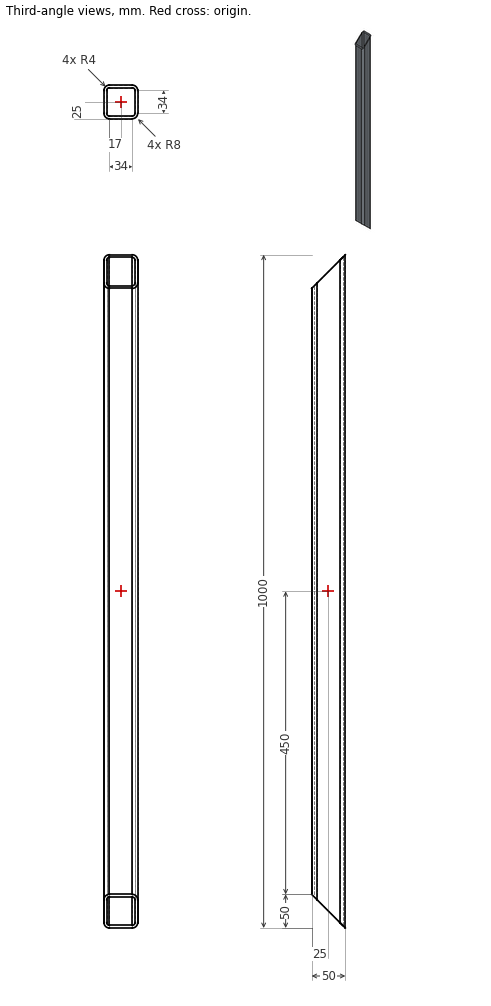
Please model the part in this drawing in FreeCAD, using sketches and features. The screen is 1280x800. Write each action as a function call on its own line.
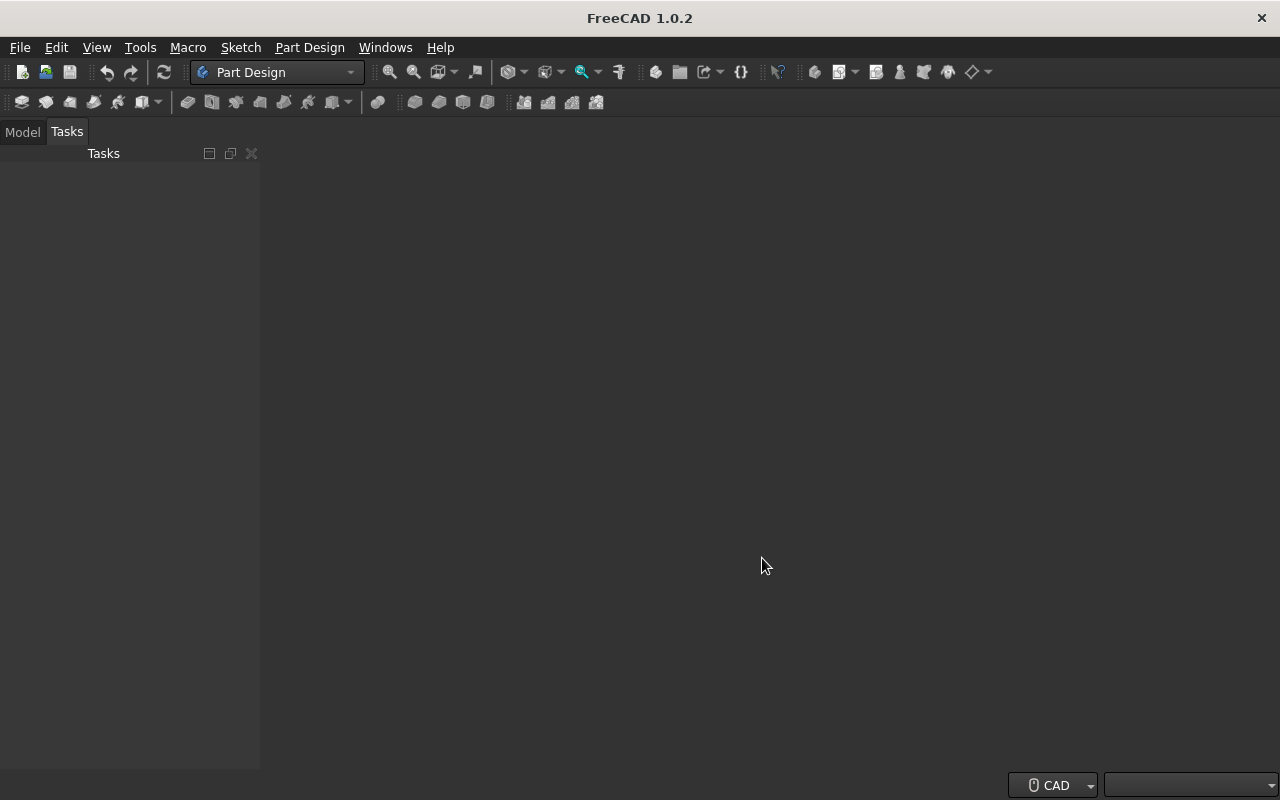
click(22, 72)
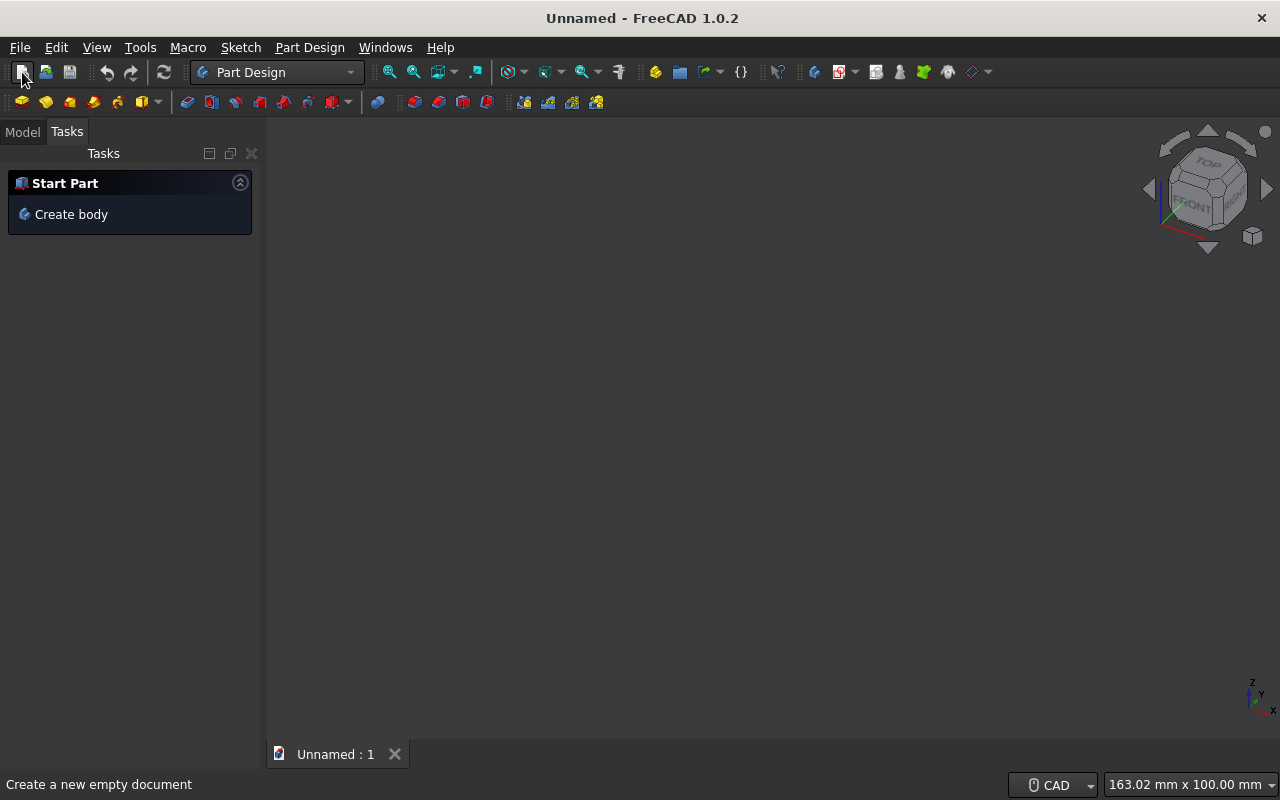
click(840, 72)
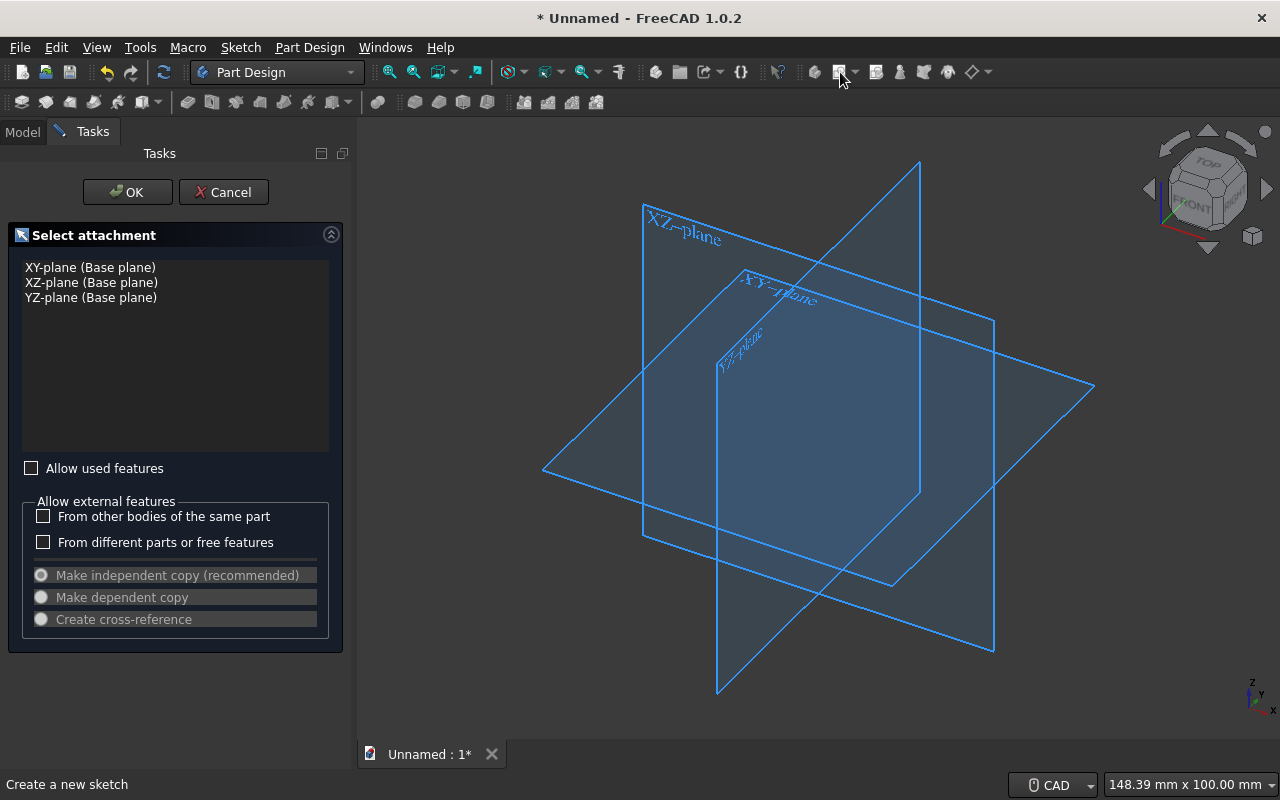
click(82, 268)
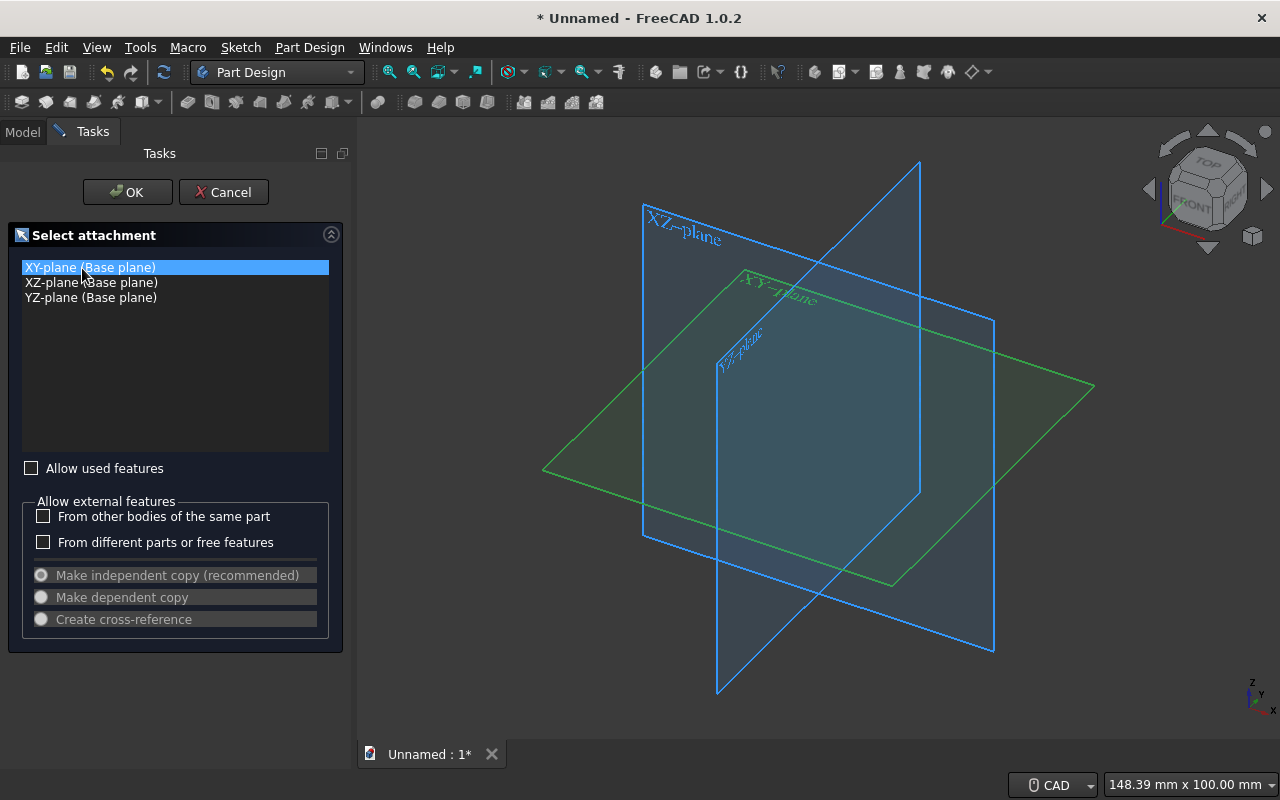
click(128, 192)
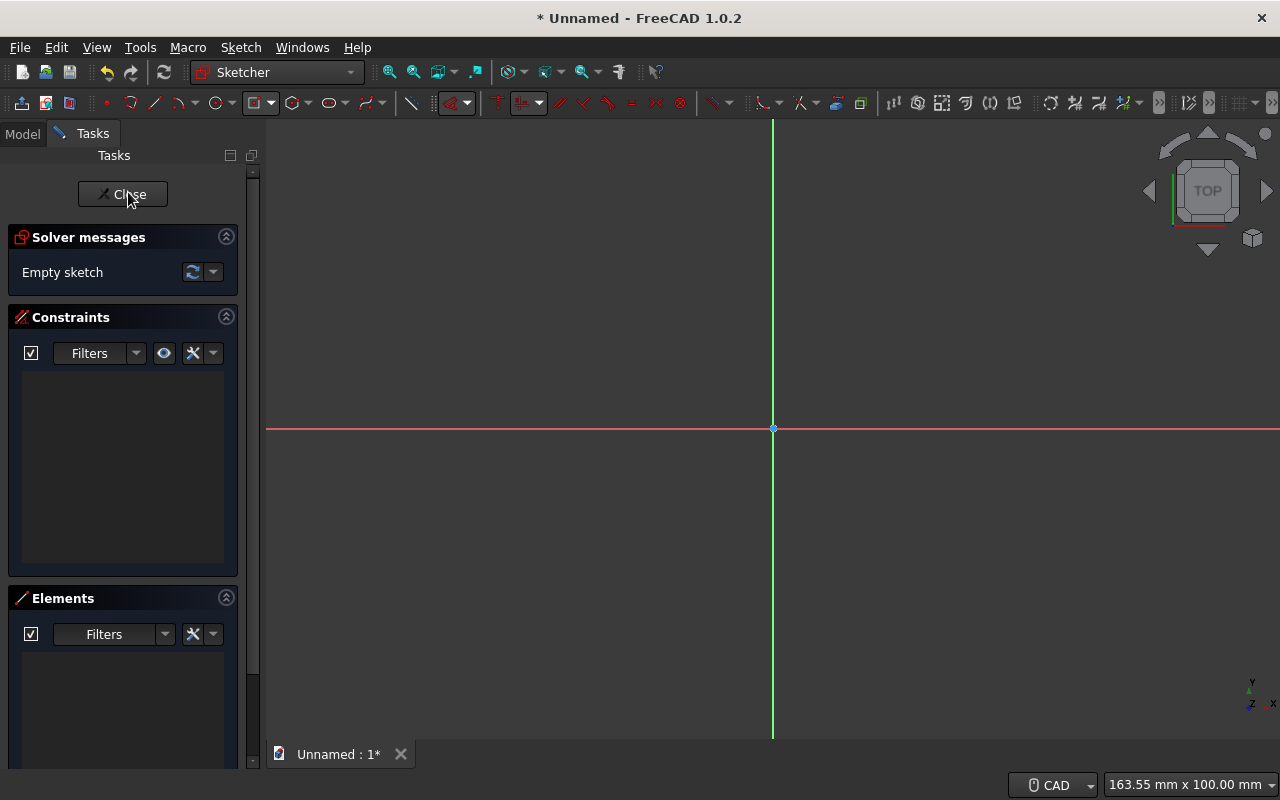
key(g)
key(l)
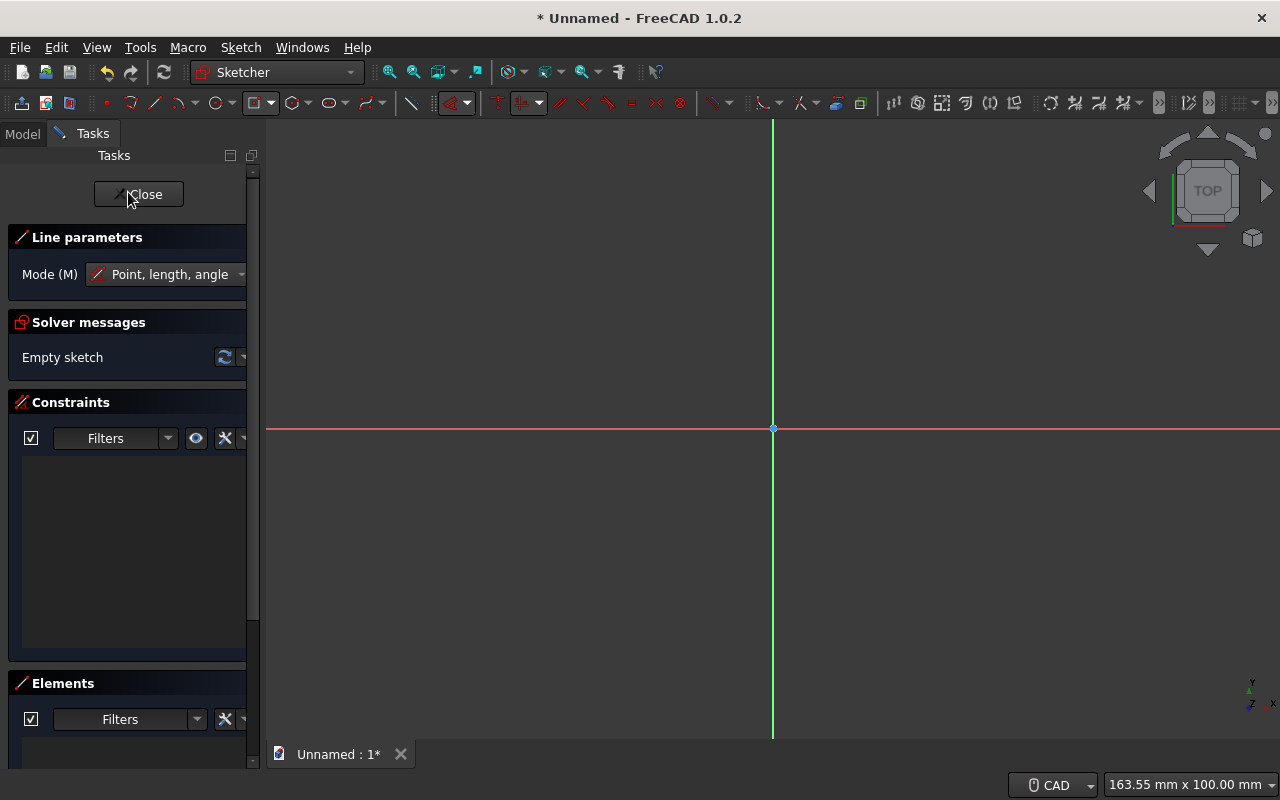
click(668, 584)
click(878, 584)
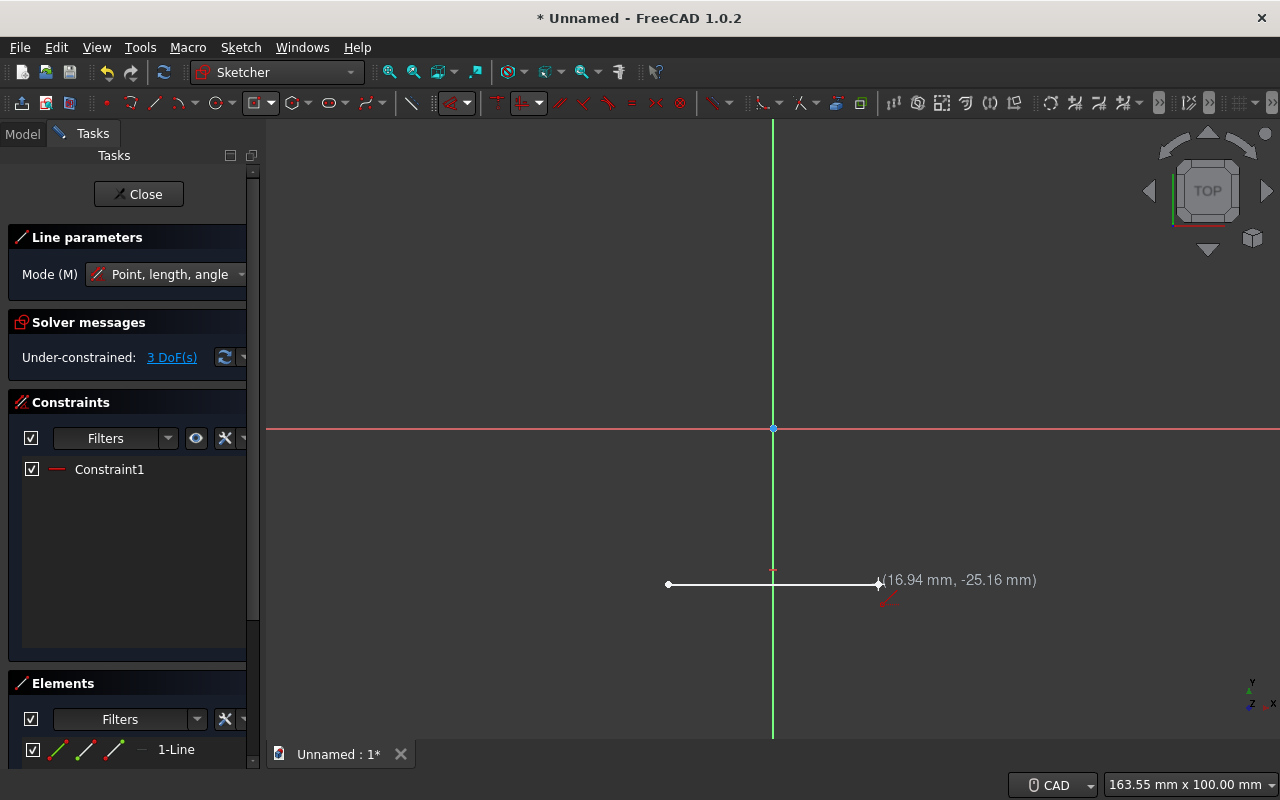
click(928, 534)
click(928, 324)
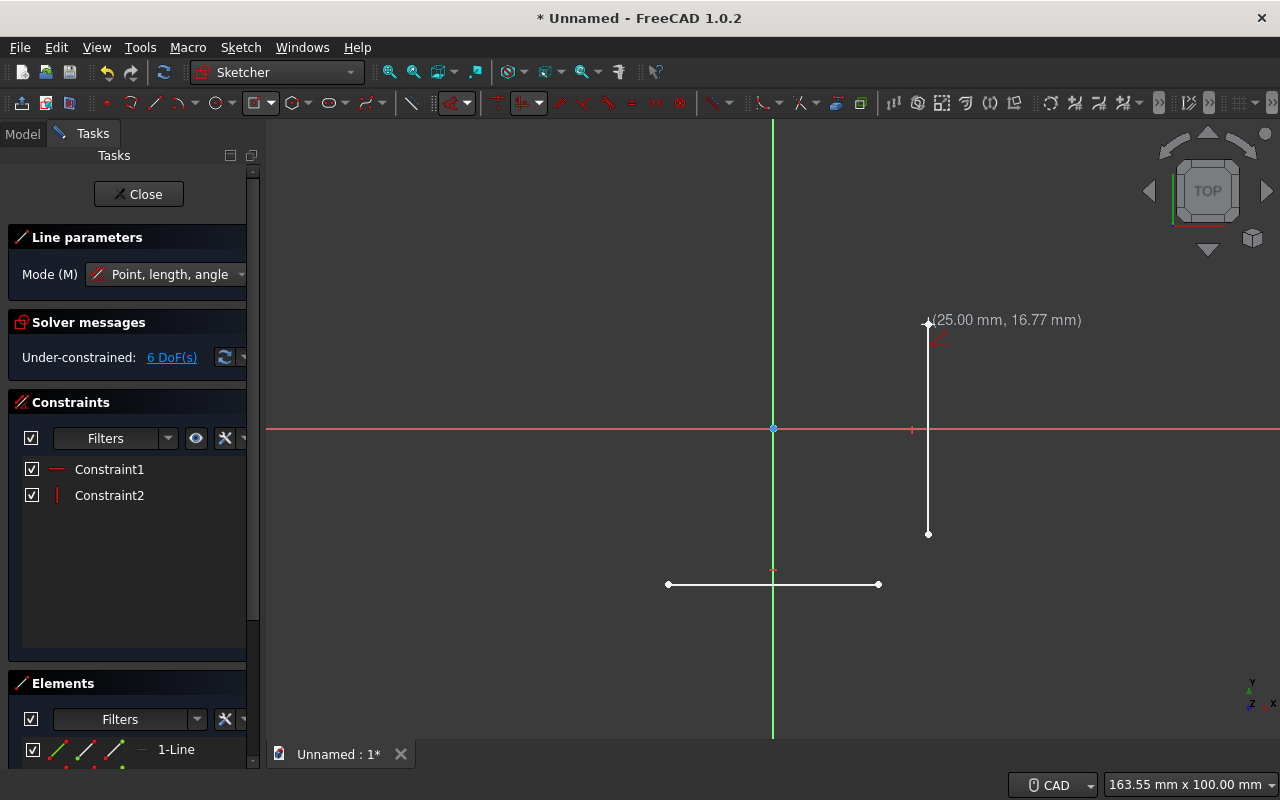
click(878, 274)
click(668, 274)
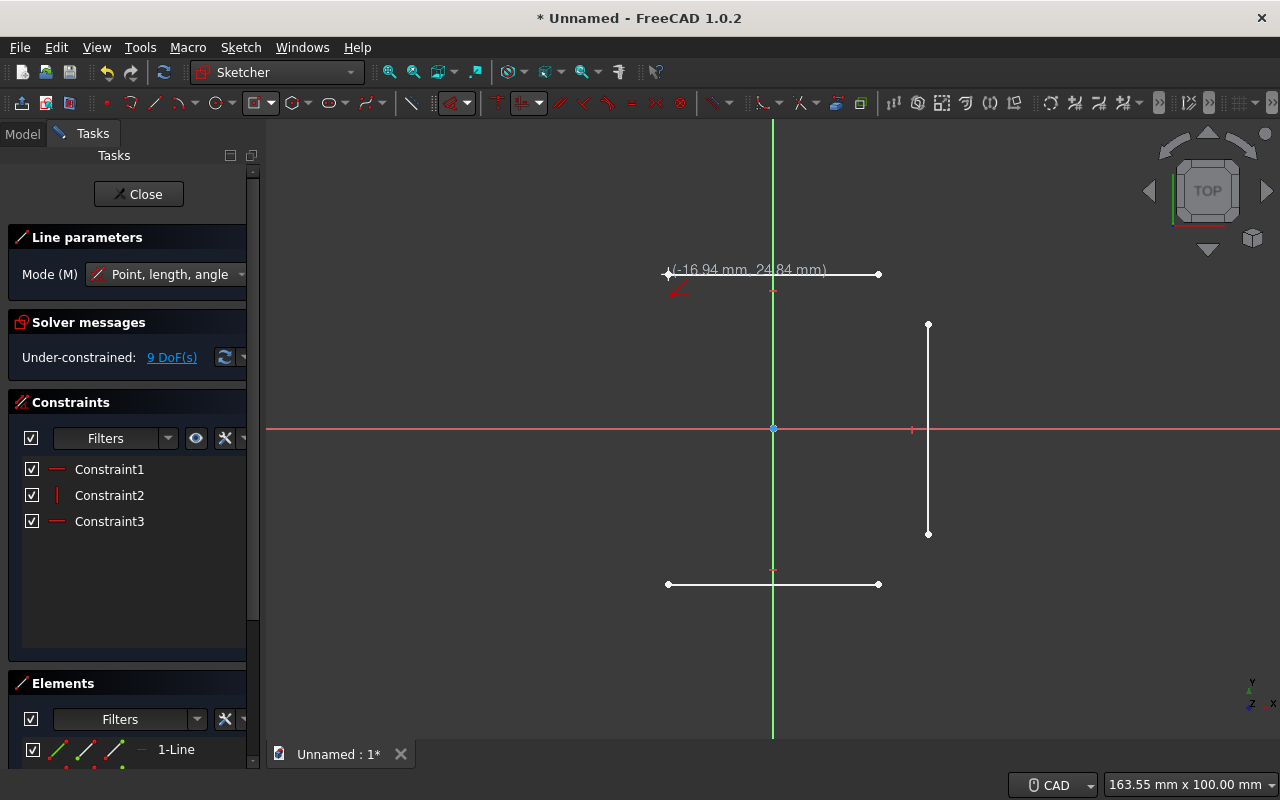
click(618, 324)
click(618, 534)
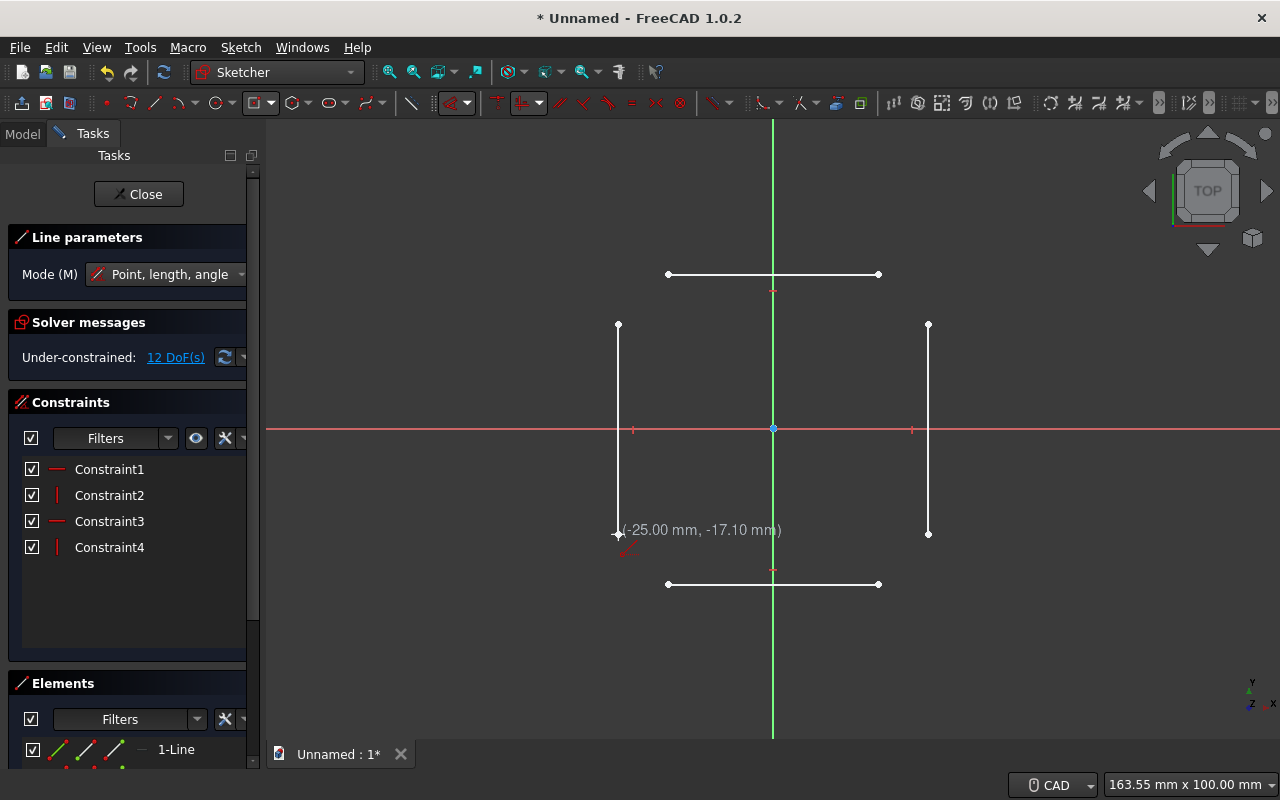
key(g)
key(3)
key(a)